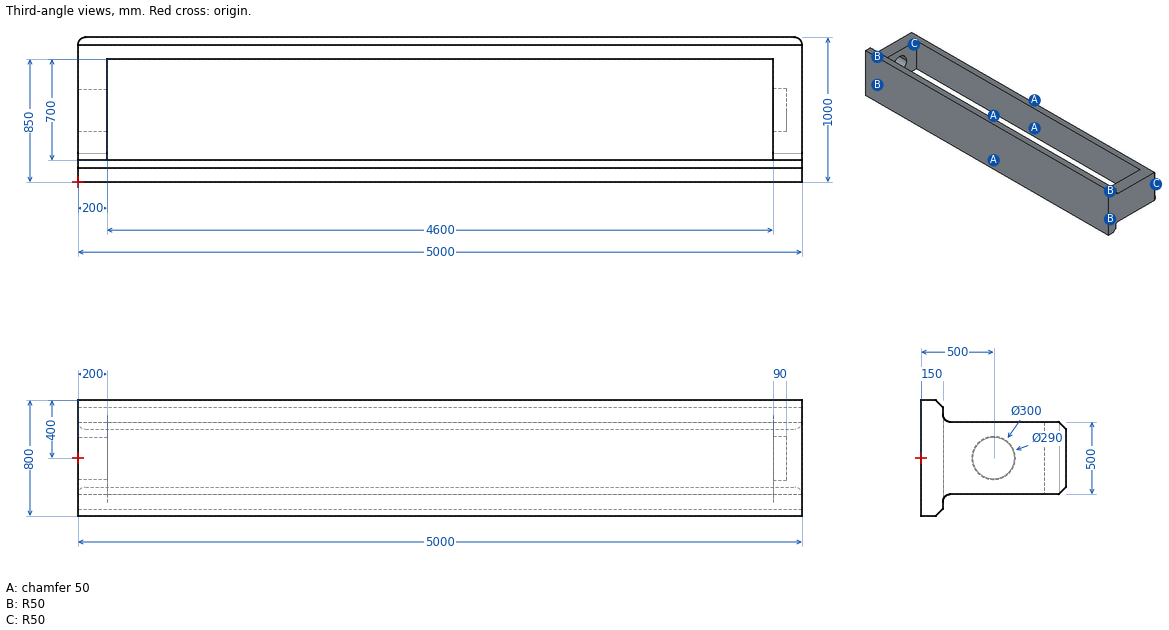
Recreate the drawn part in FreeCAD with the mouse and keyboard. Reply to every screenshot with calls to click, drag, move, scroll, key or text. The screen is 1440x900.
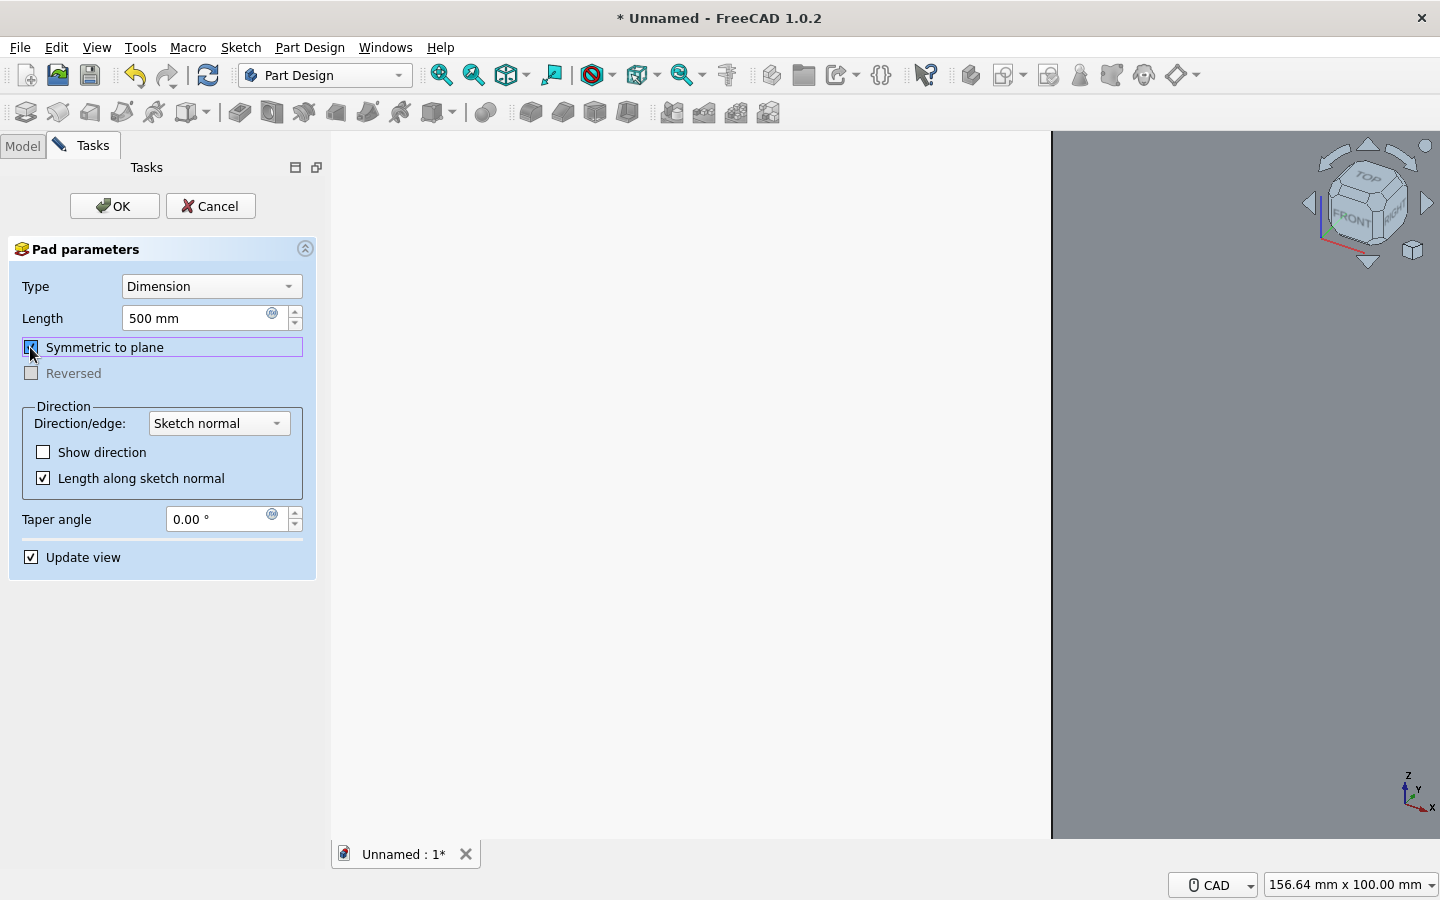
click(115, 206)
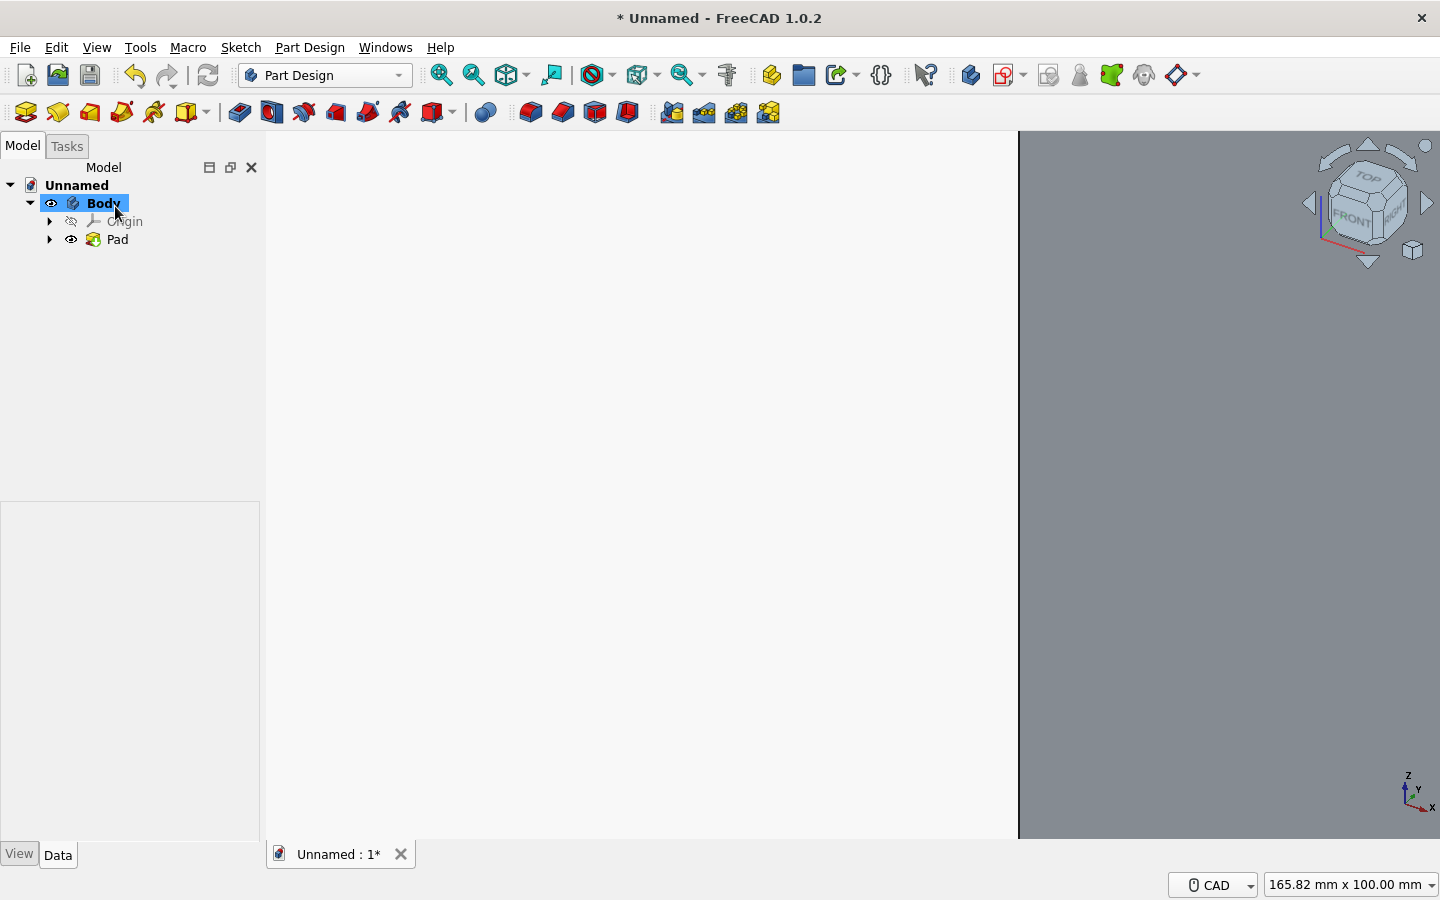
key(v)
key(f)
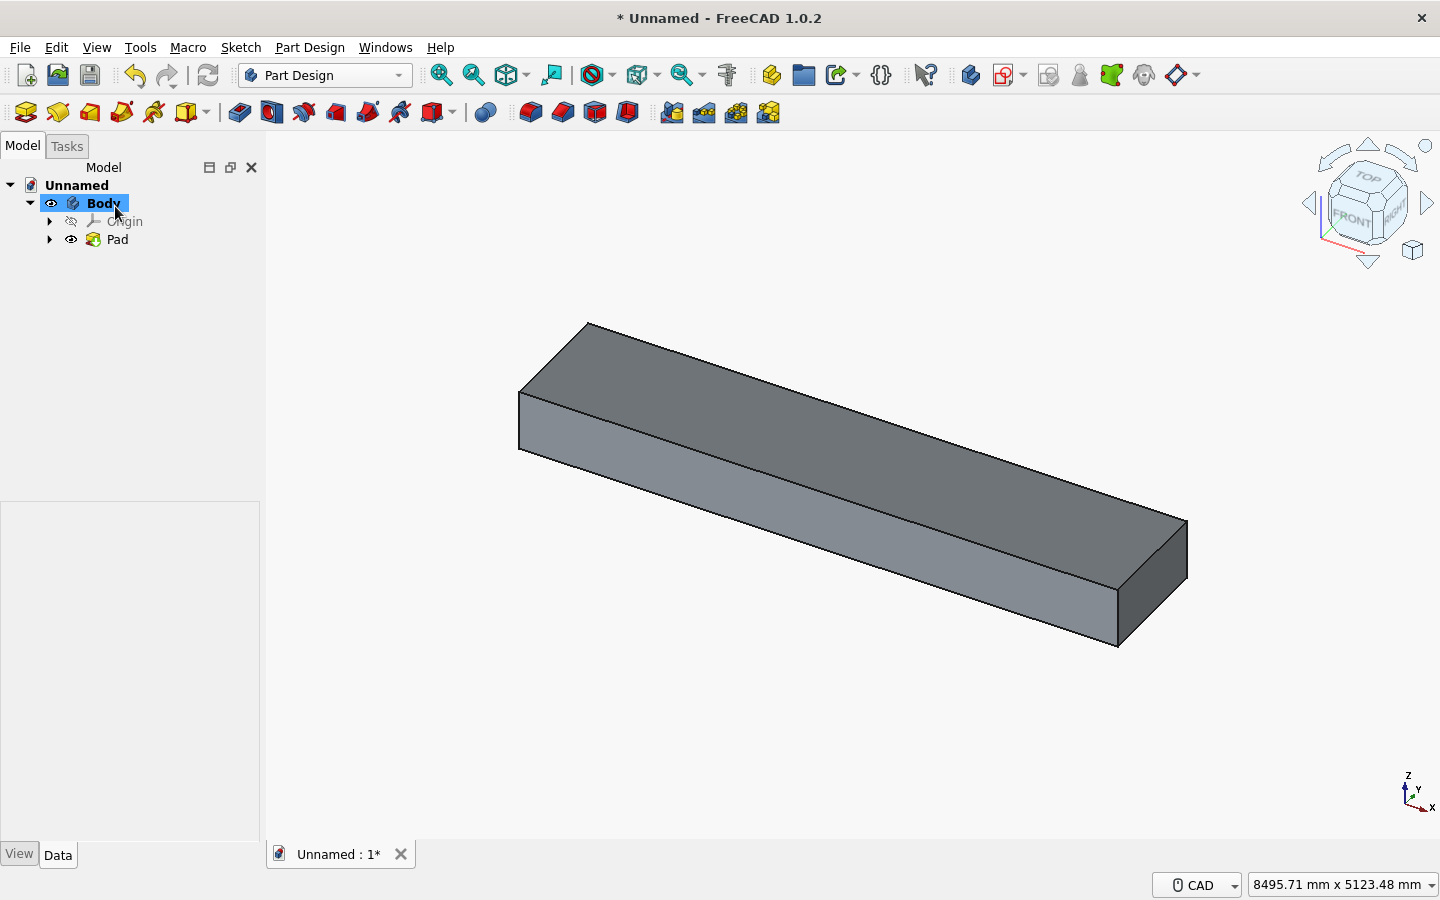
click(1024, 512)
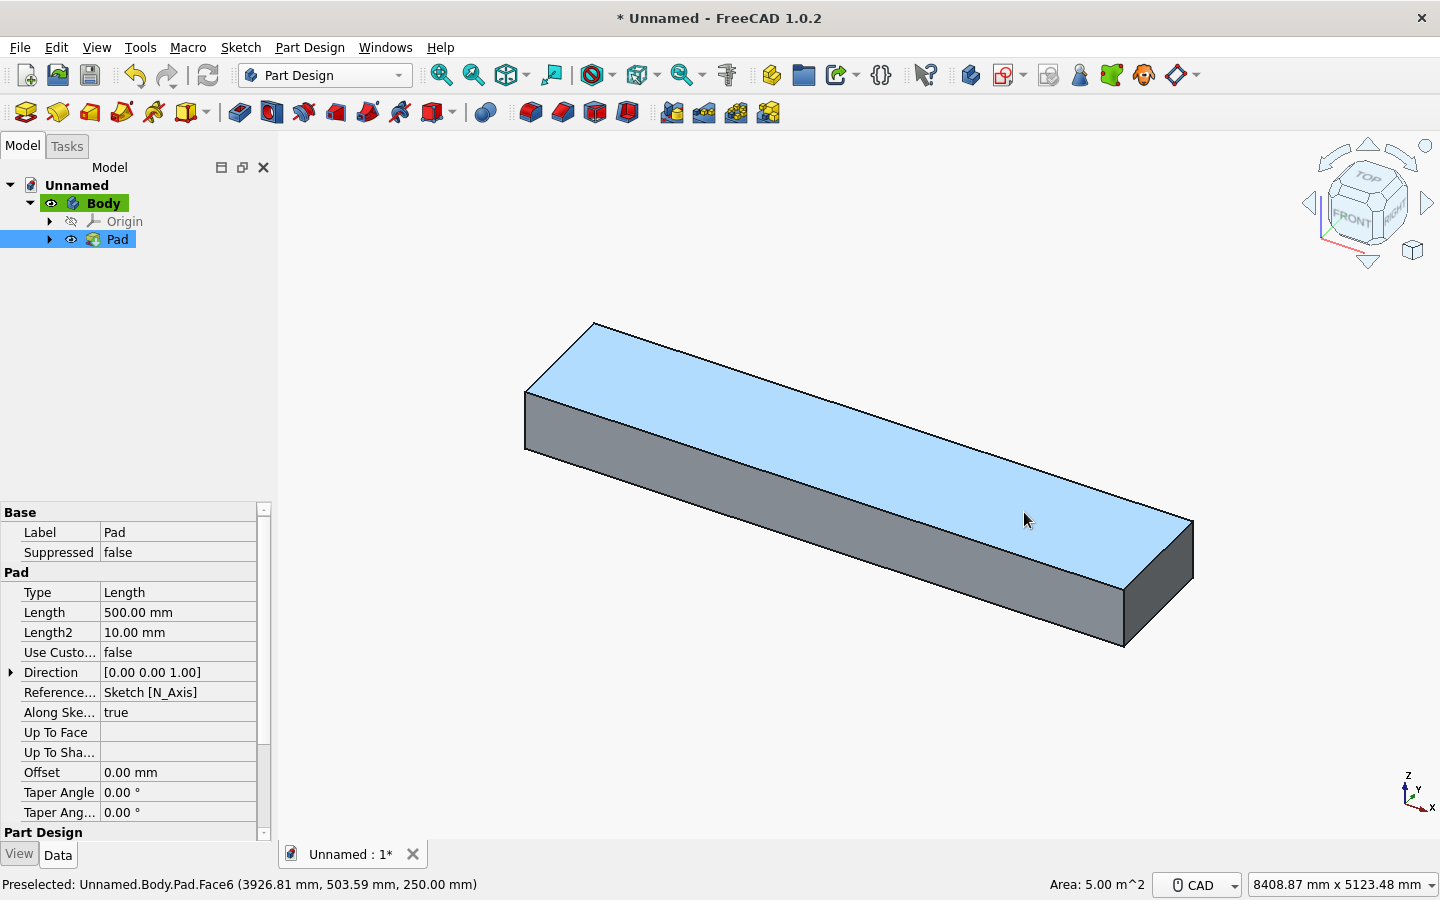
click(1004, 76)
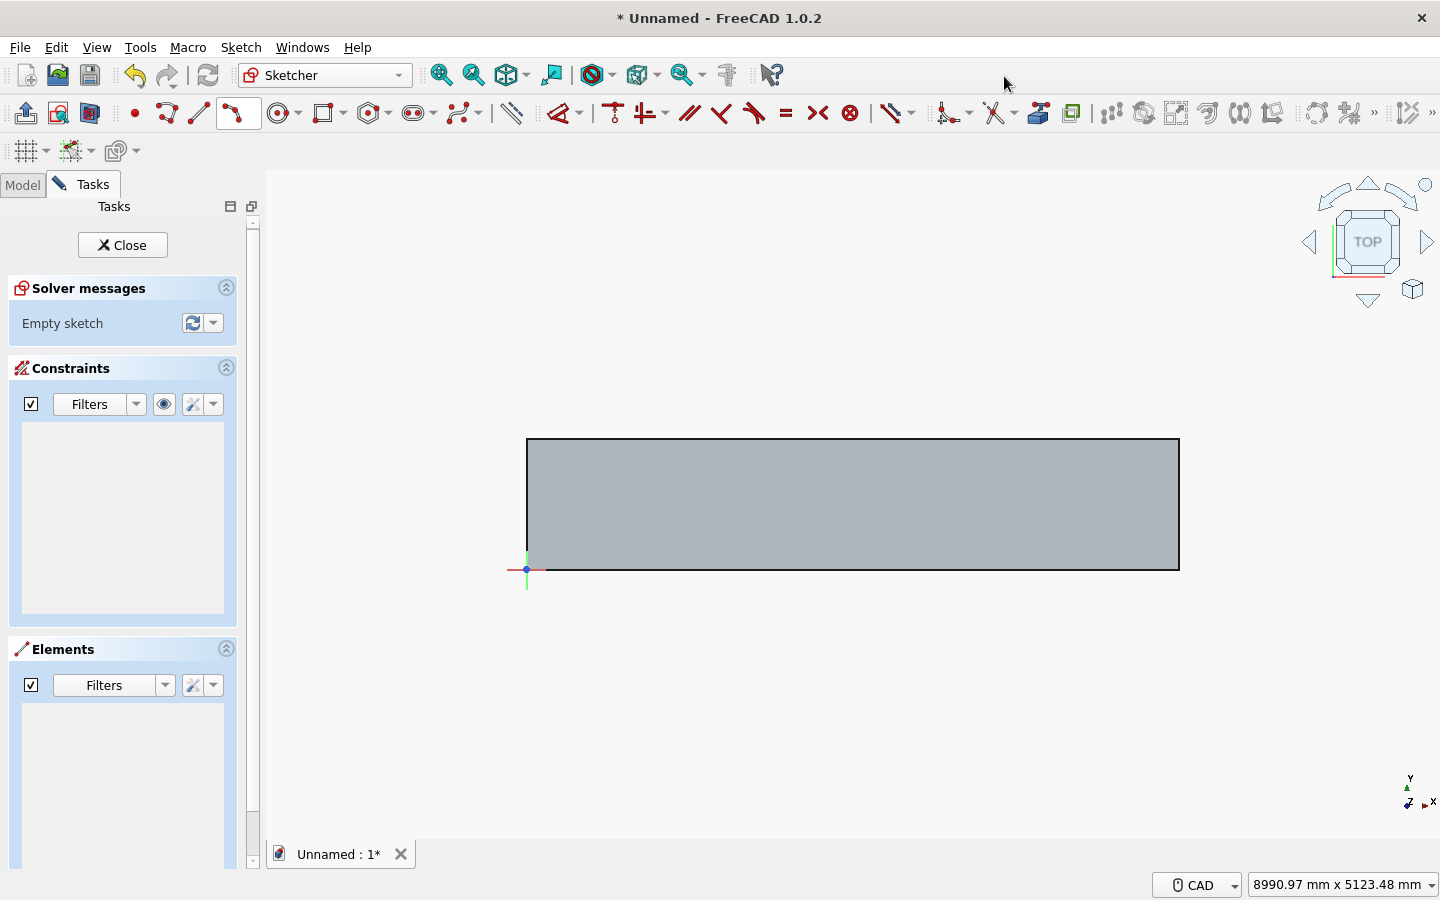
key(g)
key(r)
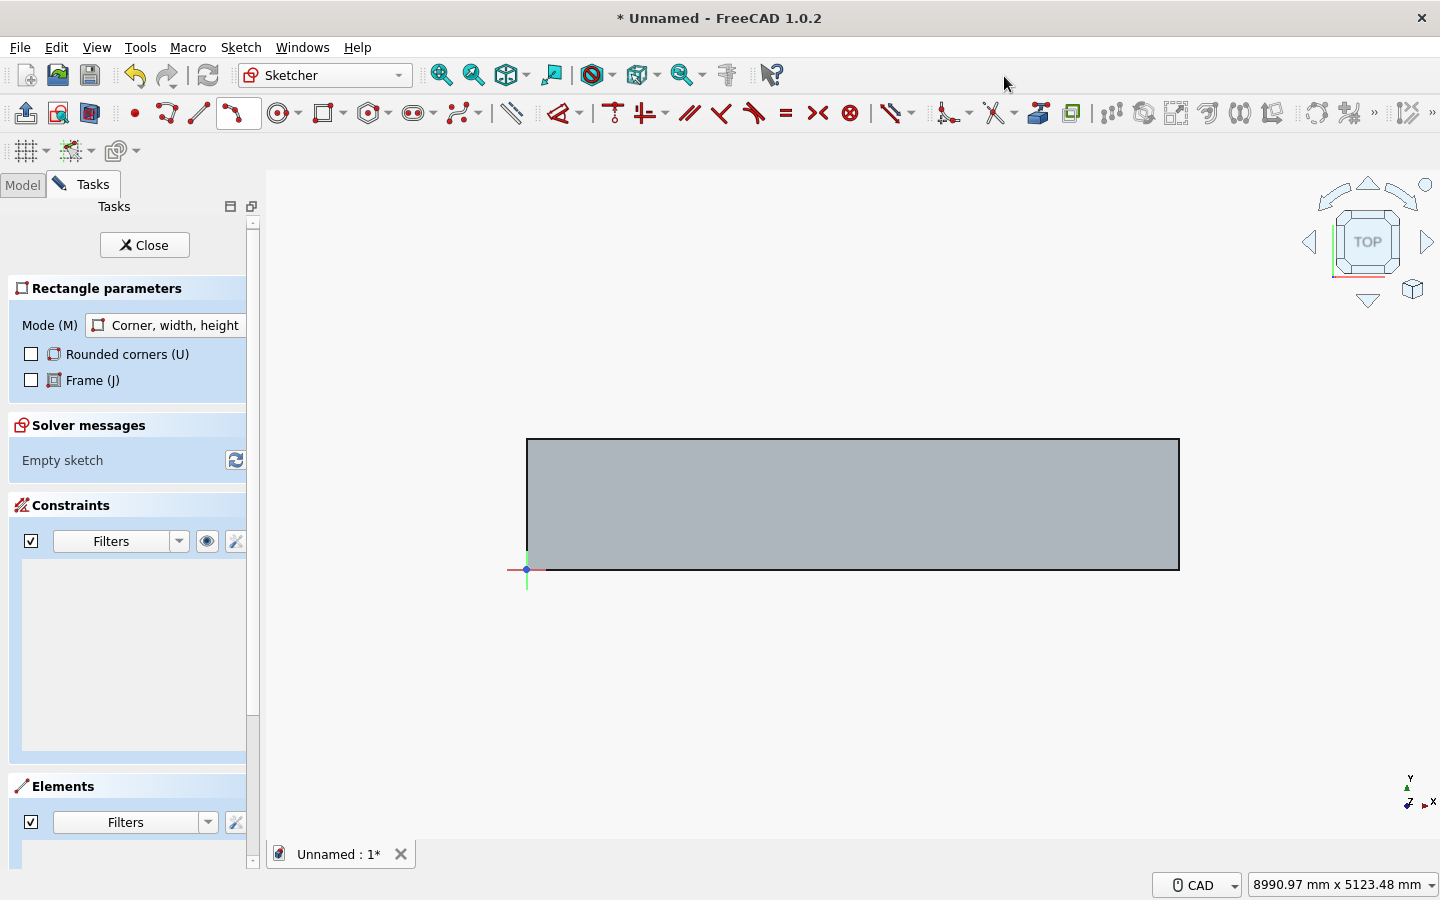
click(553, 459)
click(1153, 550)
key(Escape)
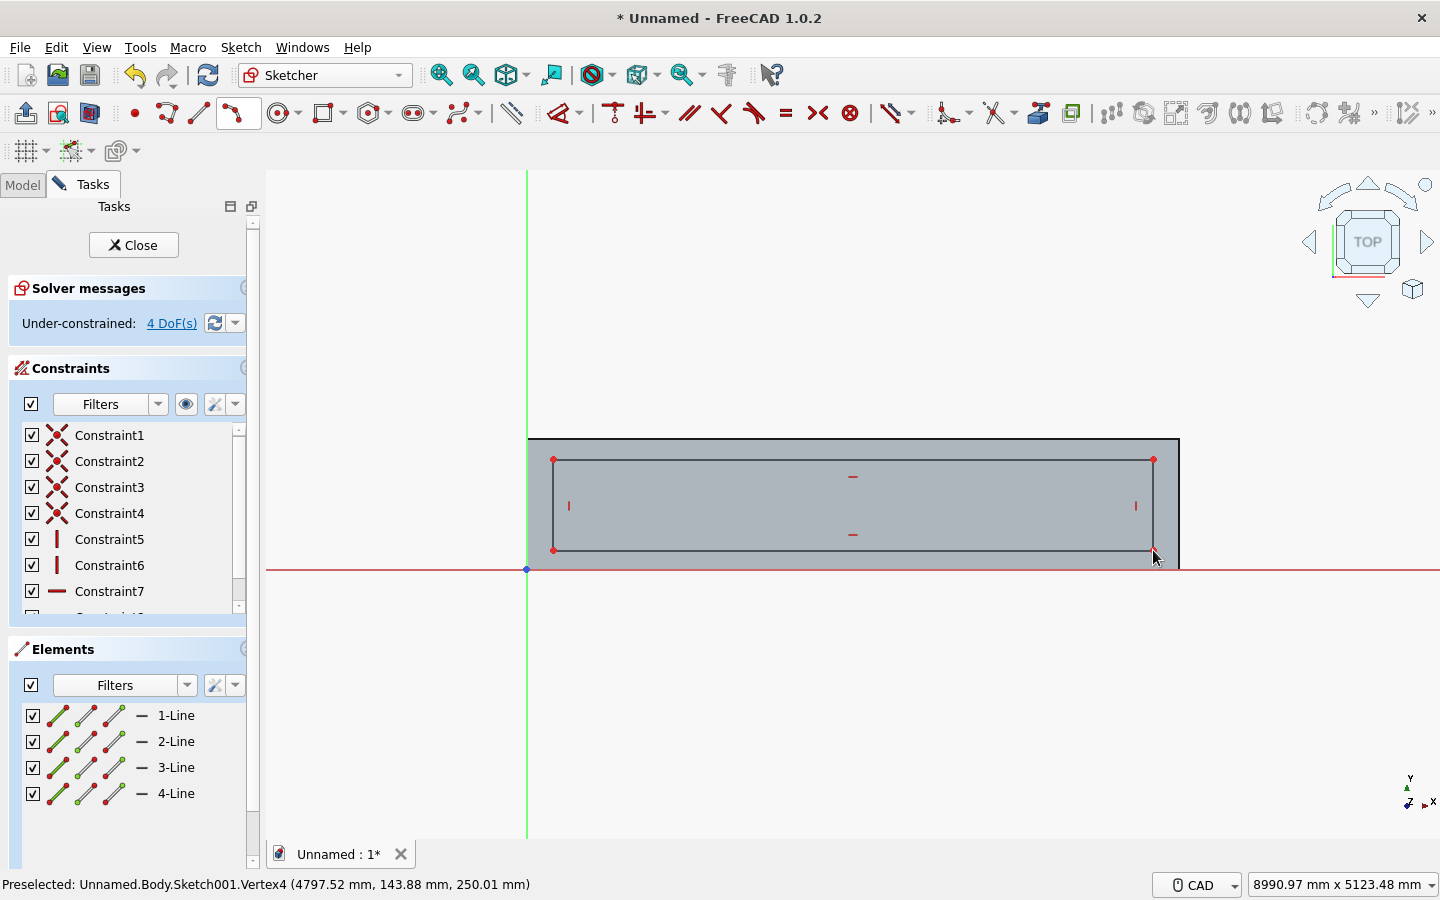
key(d)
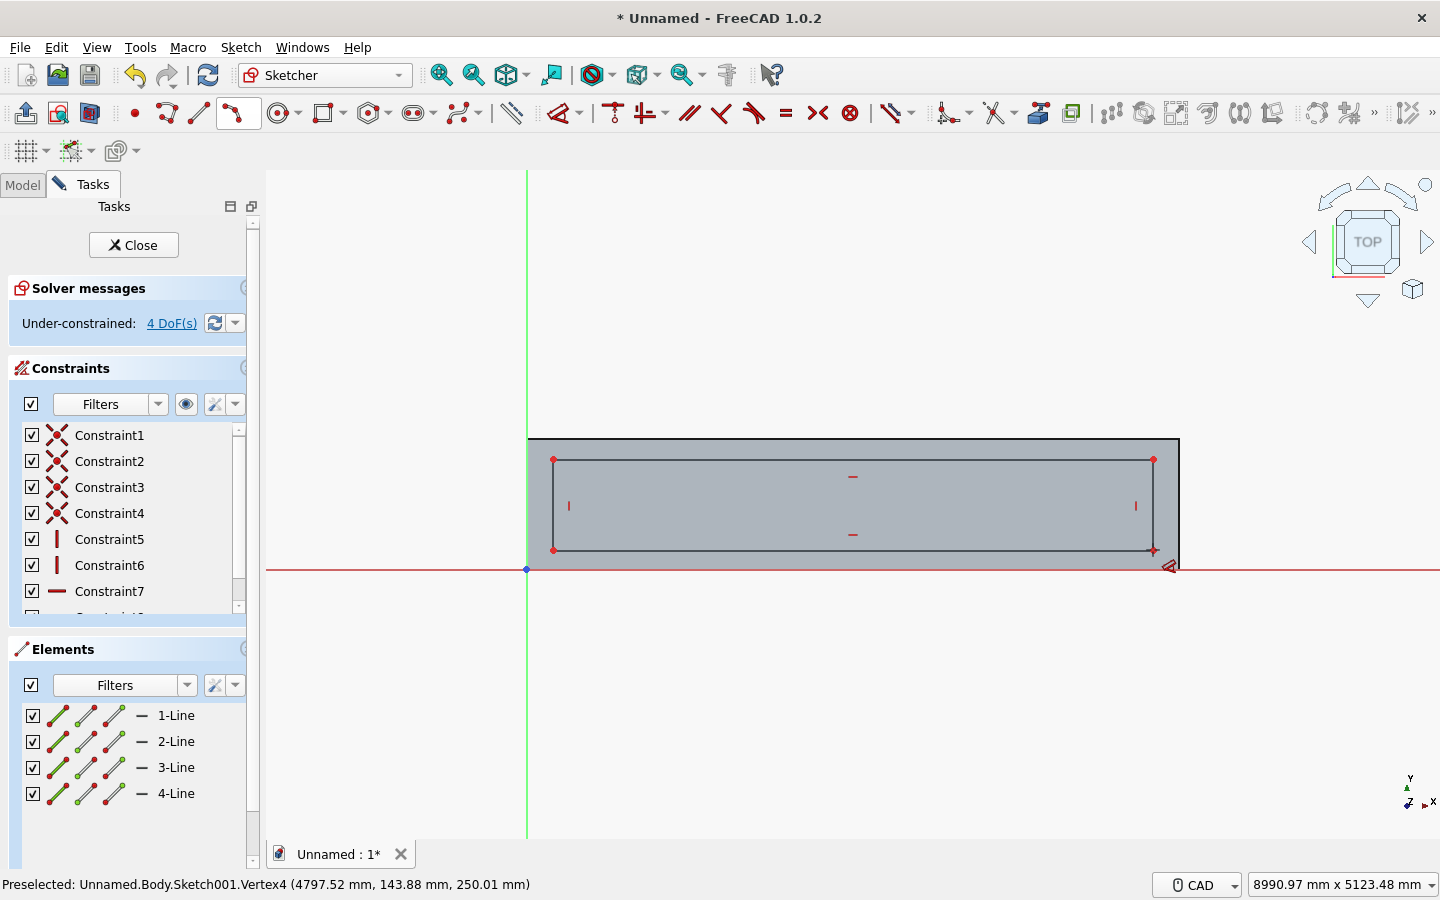
click(553, 487)
click(587, 506)